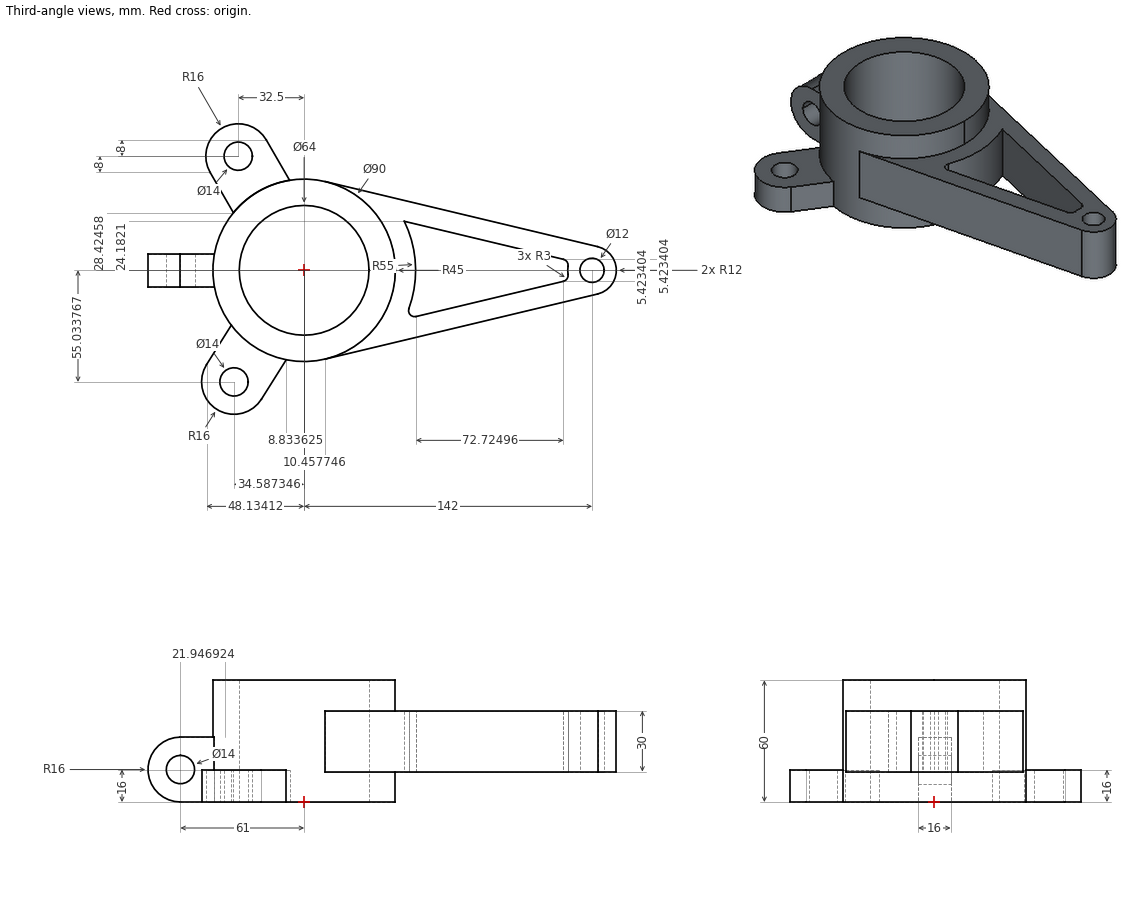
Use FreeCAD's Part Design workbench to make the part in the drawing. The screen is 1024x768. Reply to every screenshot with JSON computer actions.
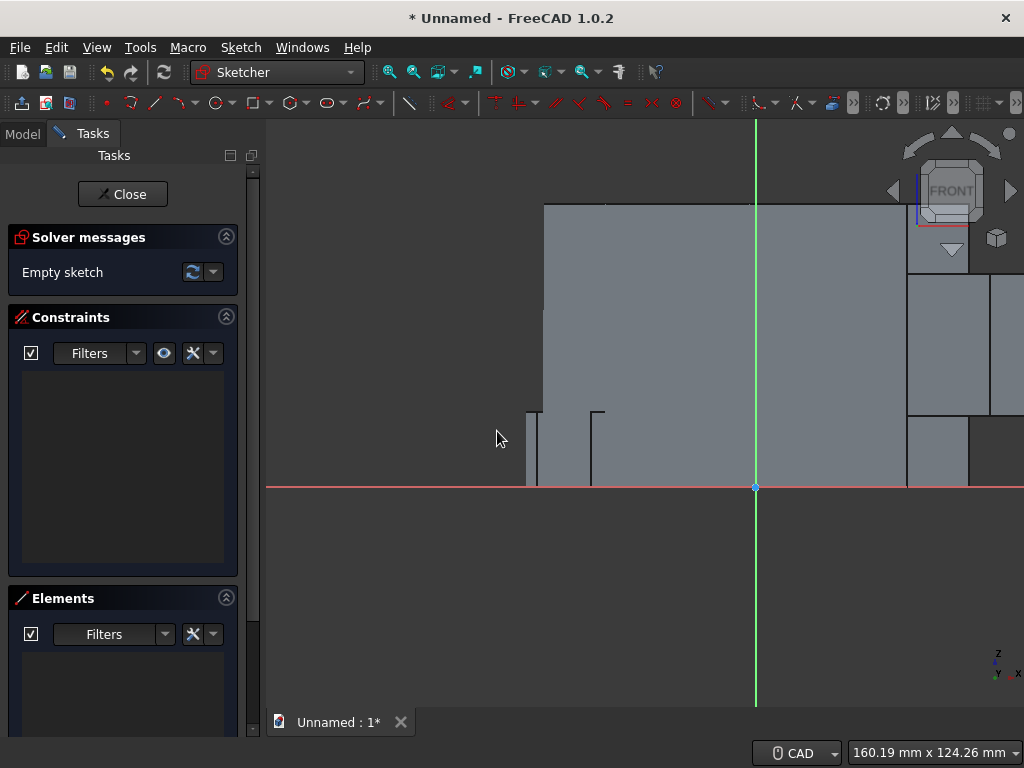
{"action": "key", "text": "g m"}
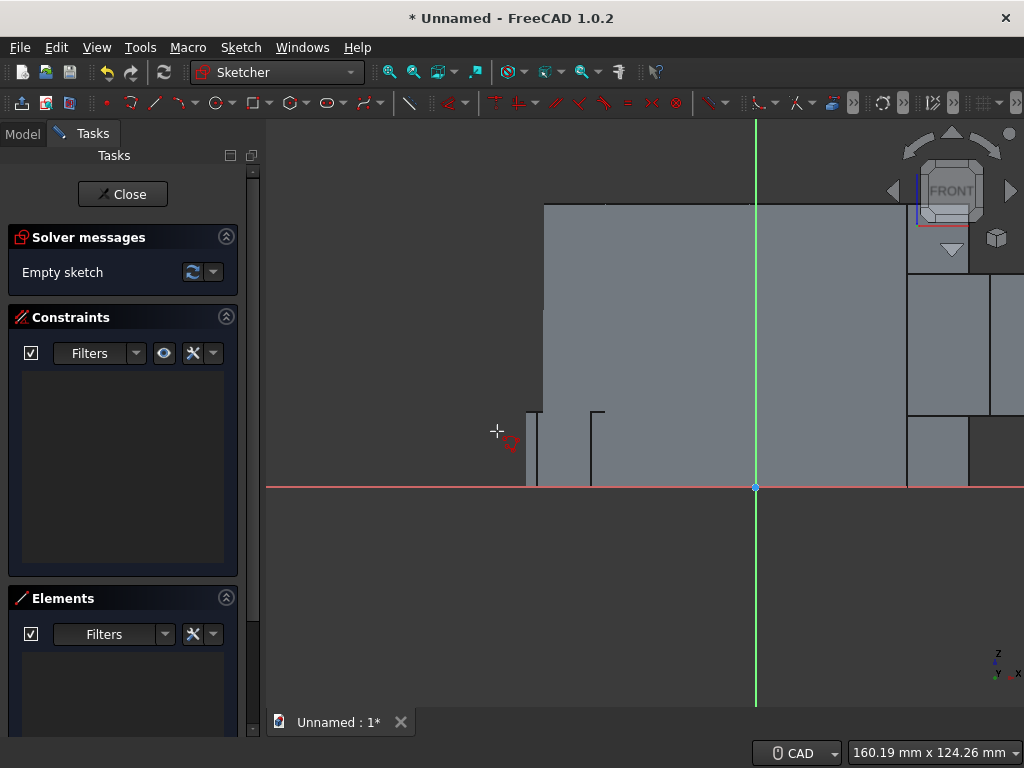
{"action": "left_click", "coordinate": [467, 336]}
{"action": "left_click", "coordinate": [571, 336]}
{"action": "left_click", "coordinate": [571, 487]}
{"action": "left_click", "coordinate": [467, 478]}
{"action": "right_click", "coordinate": [467, 478]}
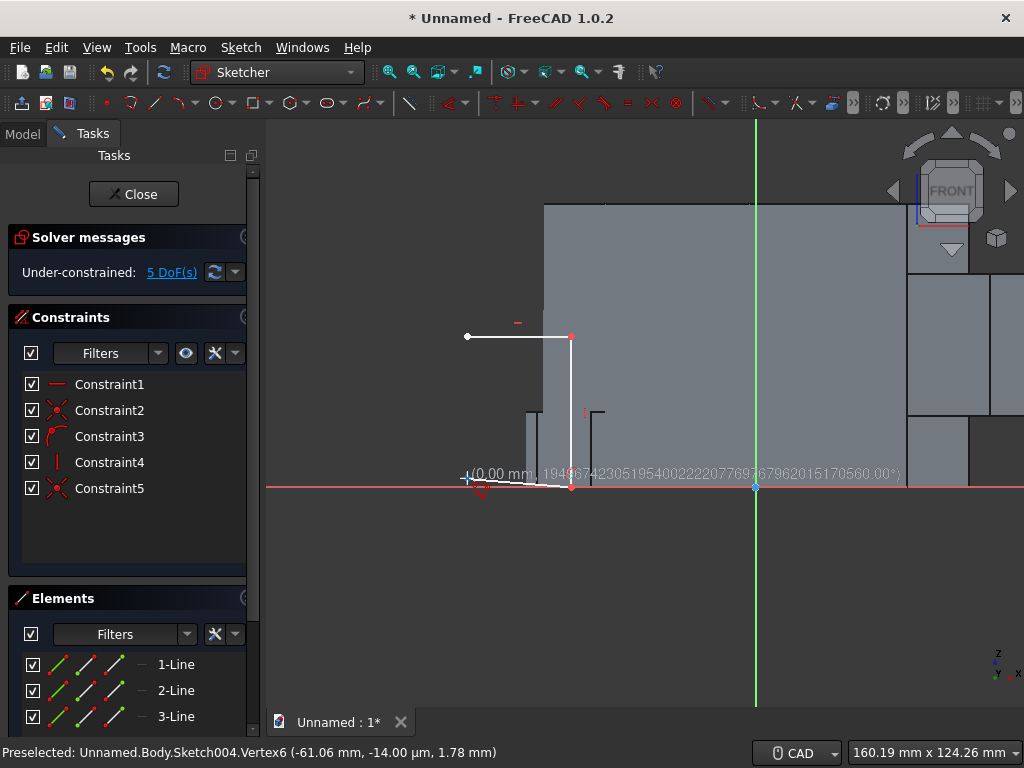
{"action": "key", "text": "g 3 a"}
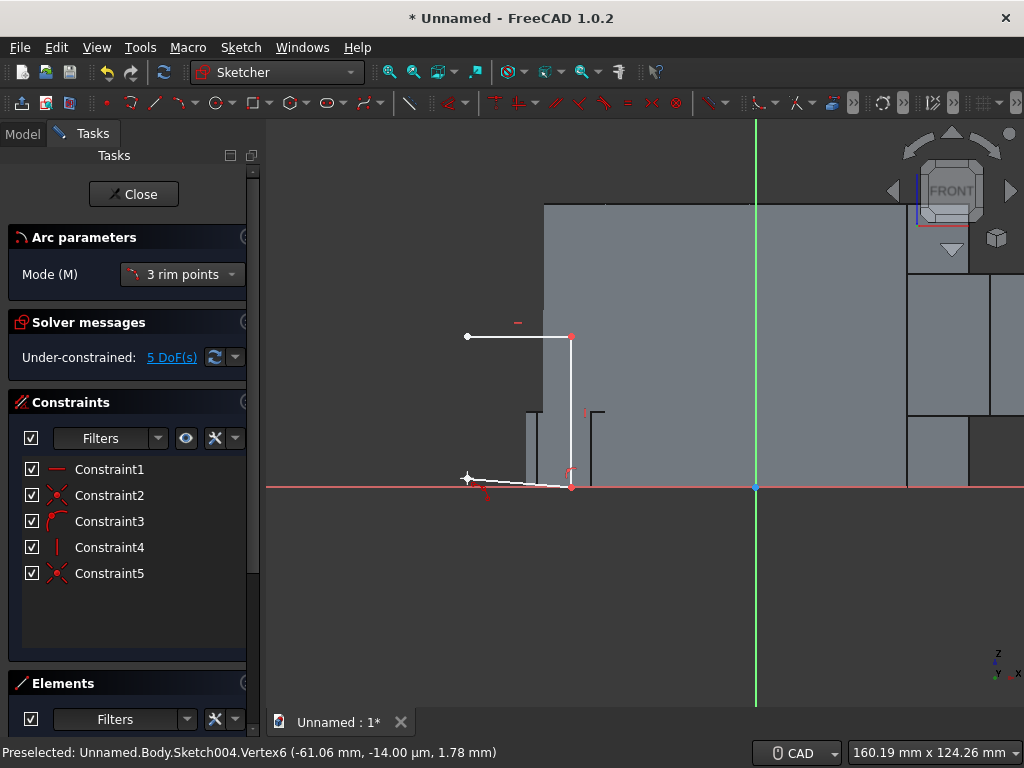
{"action": "left_click", "coordinate": [467, 479]}
{"action": "left_click", "coordinate": [467, 337]}
{"action": "left_click", "coordinate": [392, 412]}
{"action": "key", "text": "Escape"}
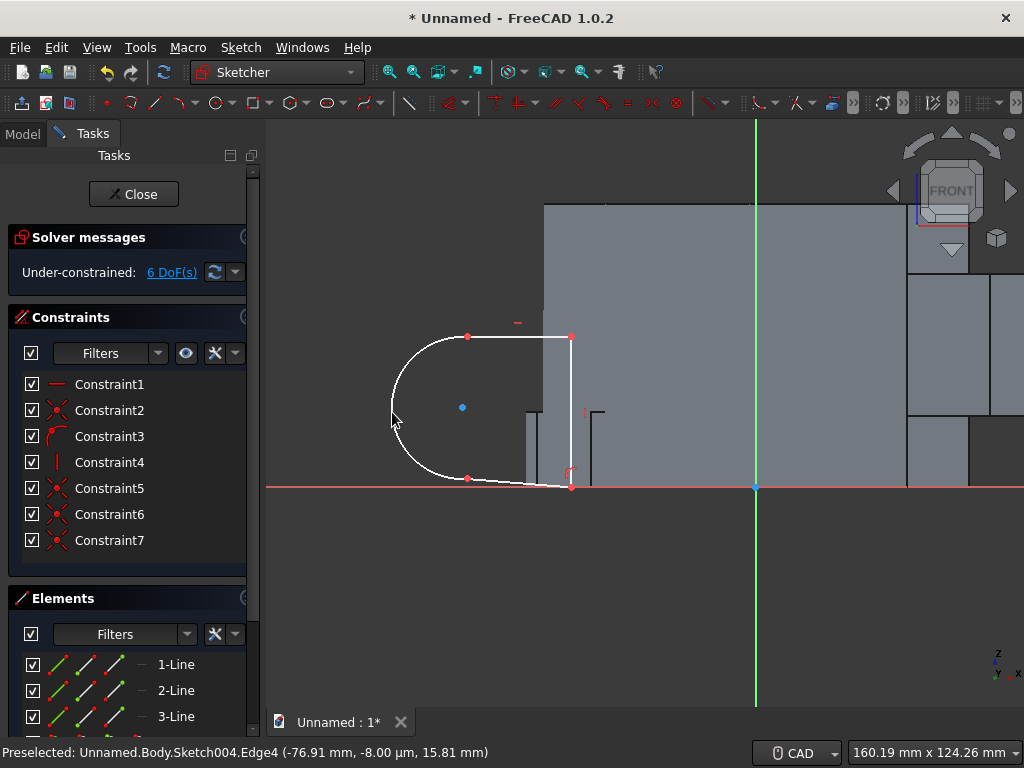
{"action": "left_click", "coordinate": [498, 337]}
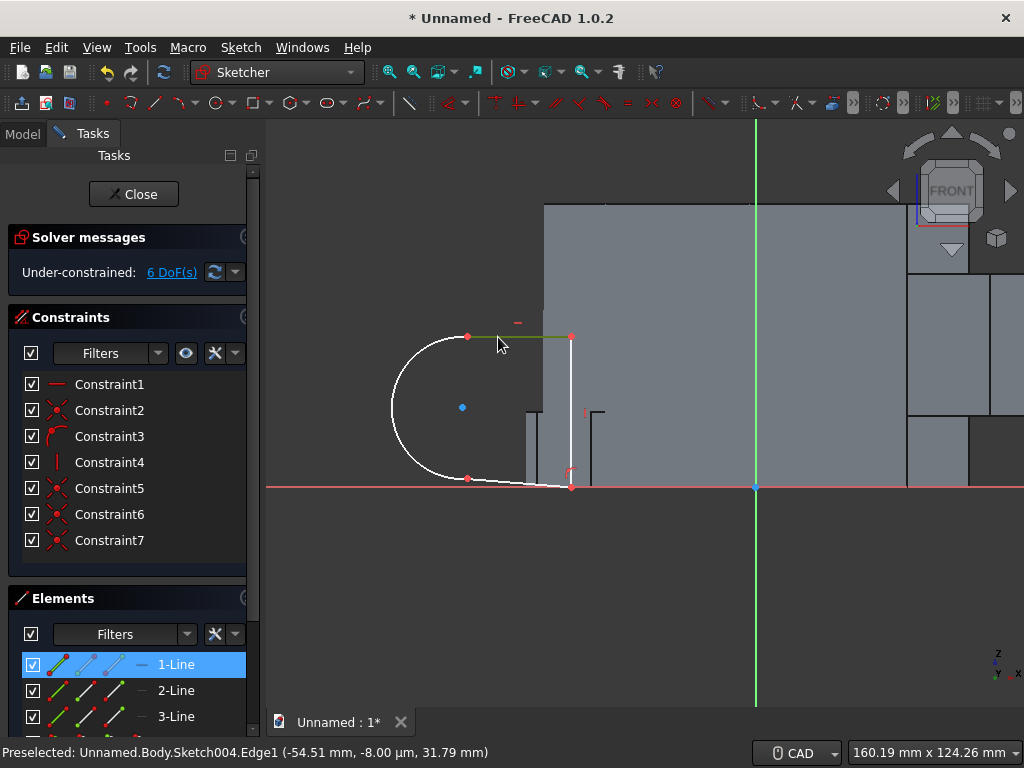
{"action": "left_click", "coordinate": [406, 365]}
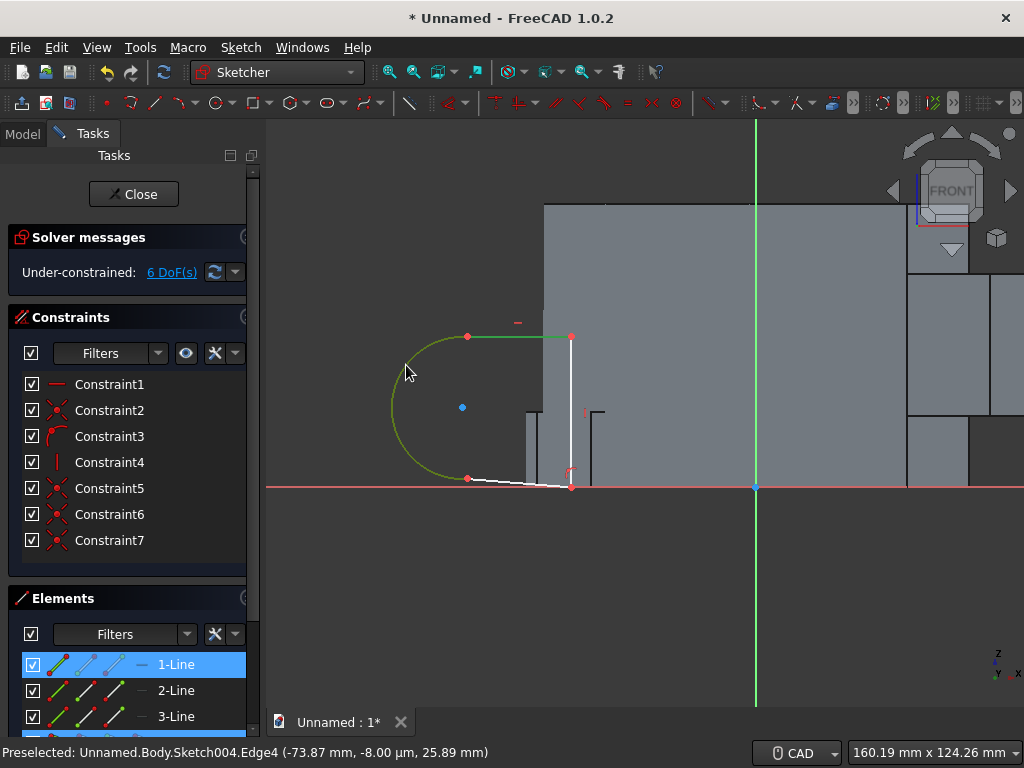
{"action": "left_click", "coordinate": [604, 104]}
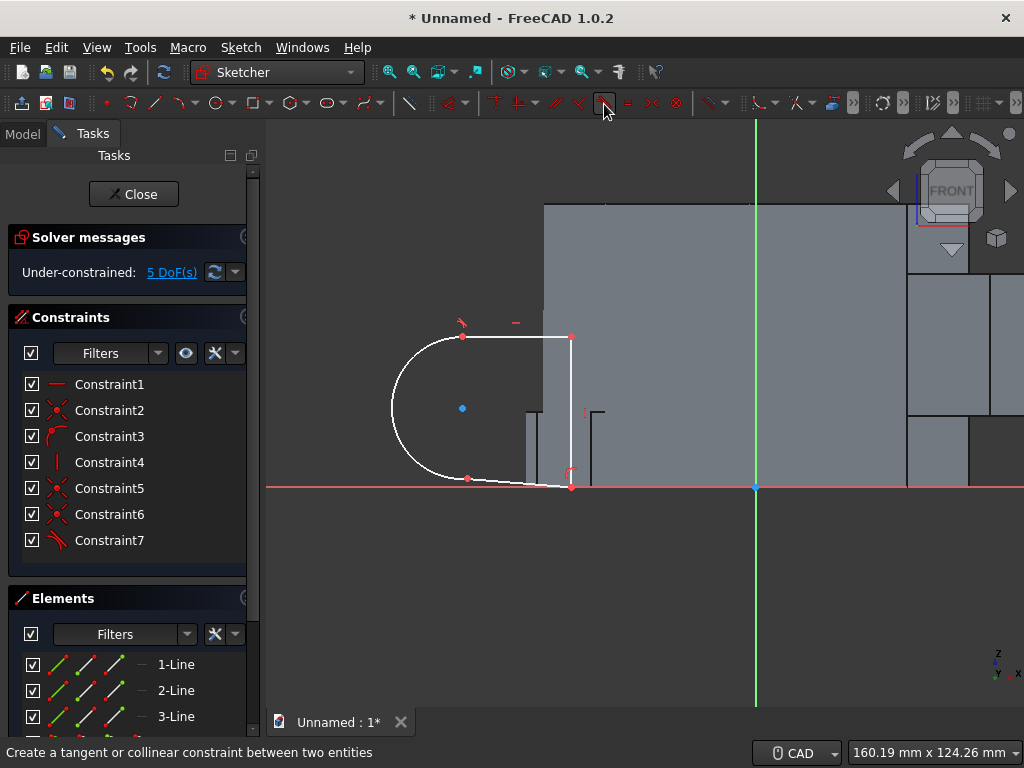
{"action": "left_click", "coordinate": [540, 485]}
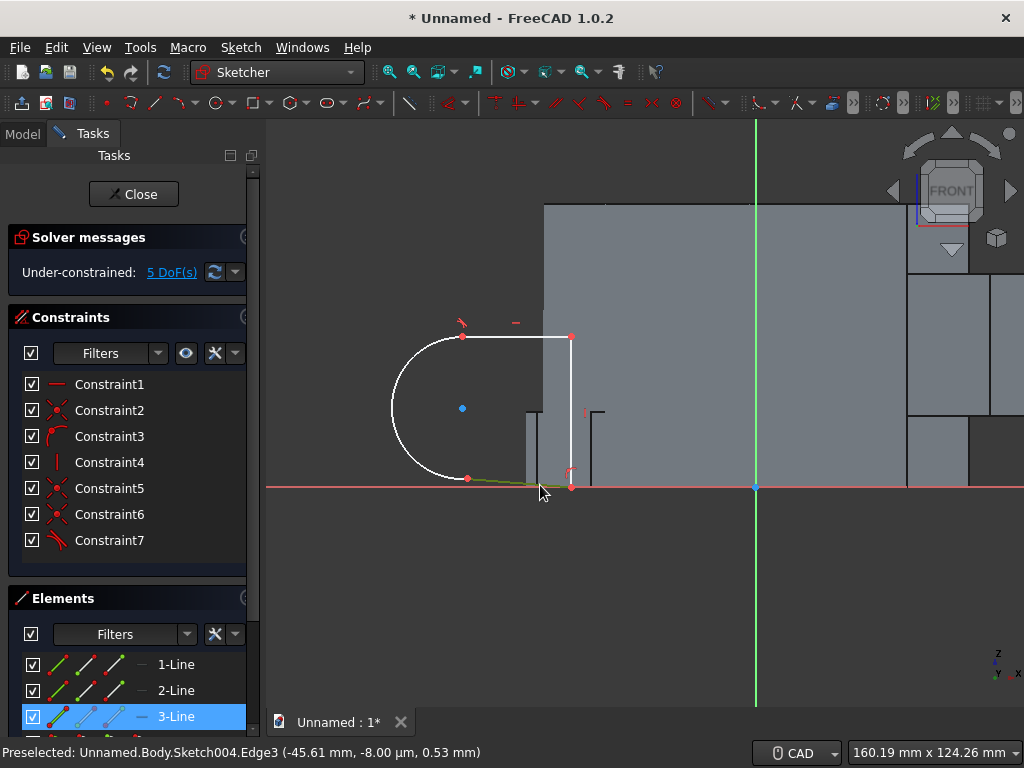
{"action": "left_click", "coordinate": [405, 367]}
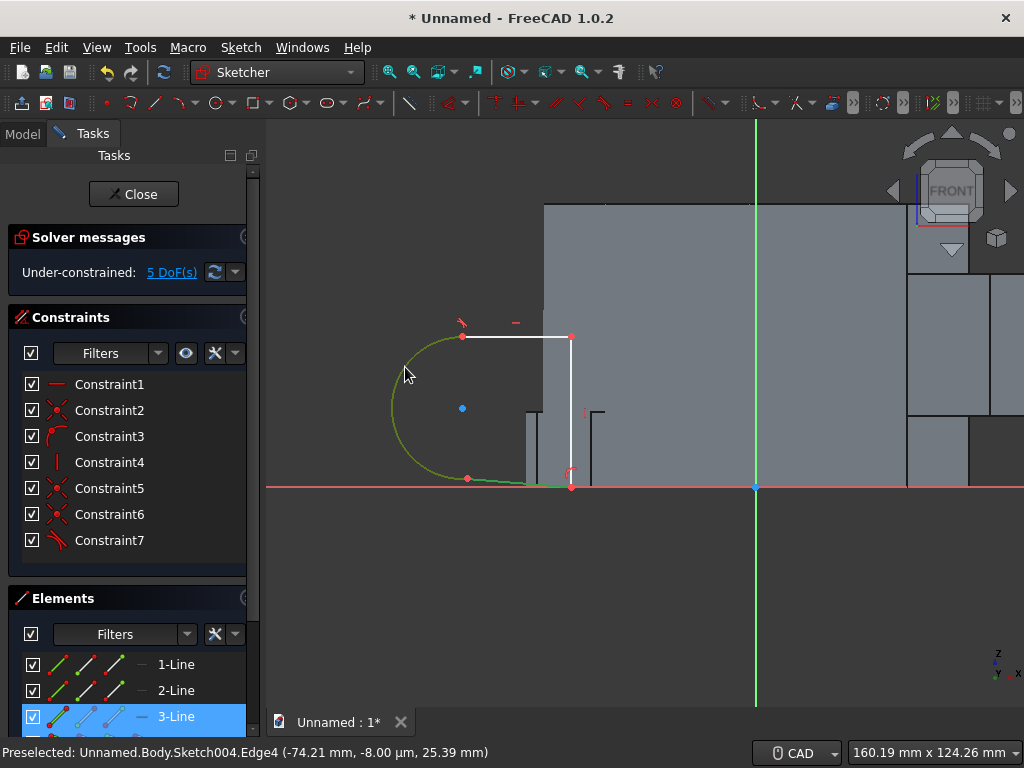
{"action": "left_click", "coordinate": [604, 104]}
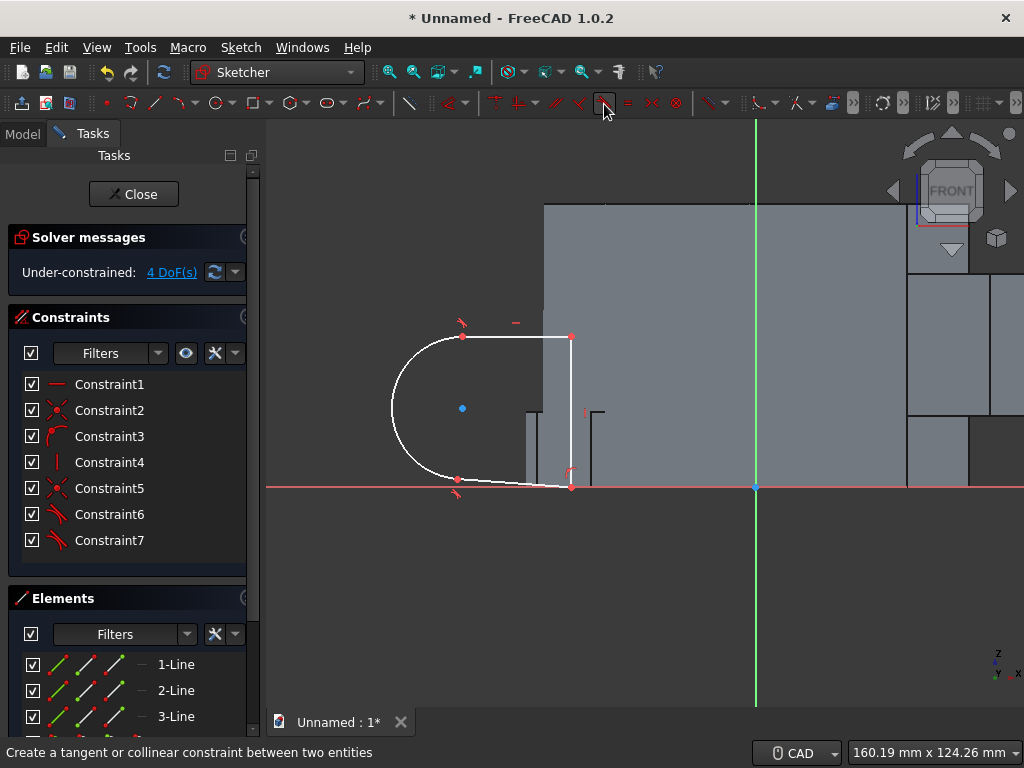
{"action": "left_click", "coordinate": [537, 485]}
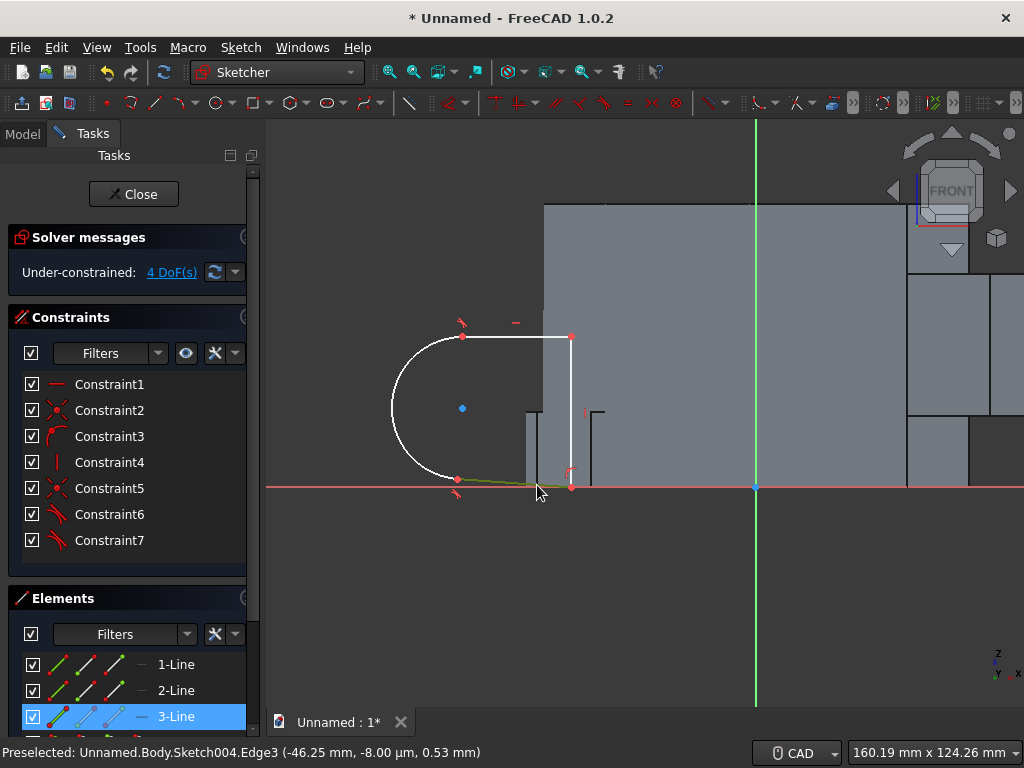
{"action": "key", "text": "h"}